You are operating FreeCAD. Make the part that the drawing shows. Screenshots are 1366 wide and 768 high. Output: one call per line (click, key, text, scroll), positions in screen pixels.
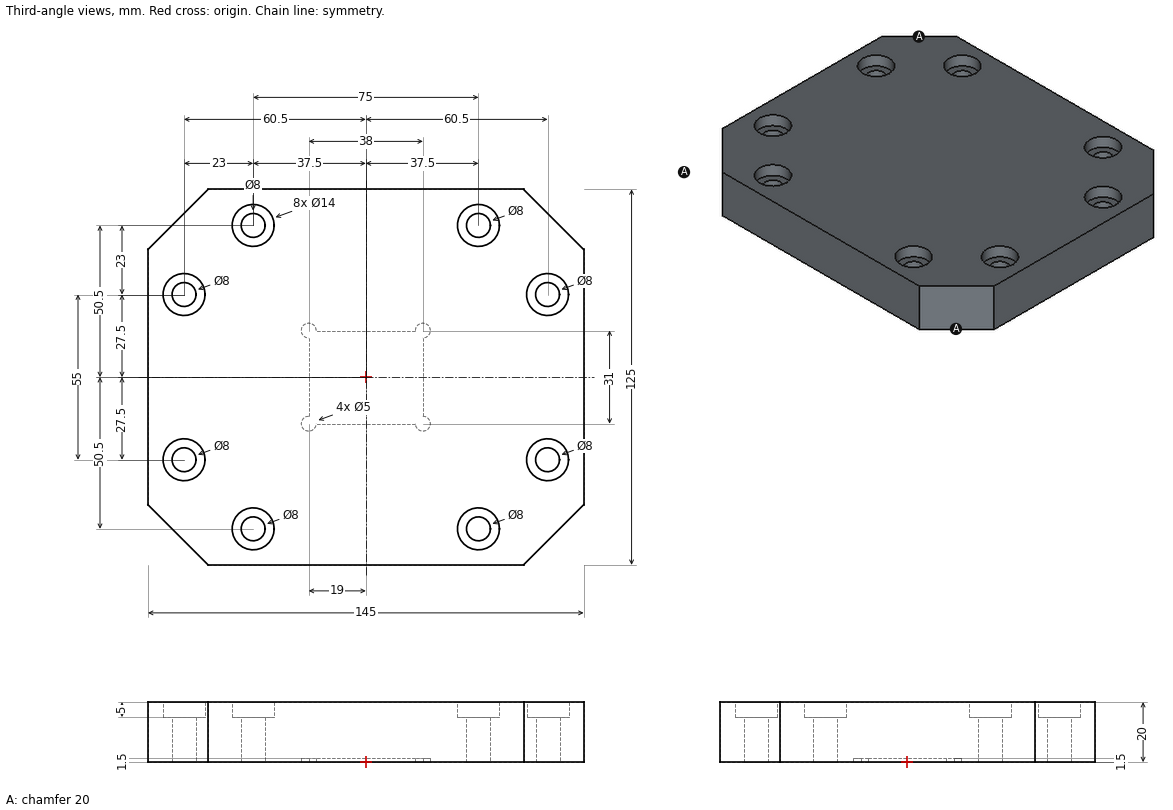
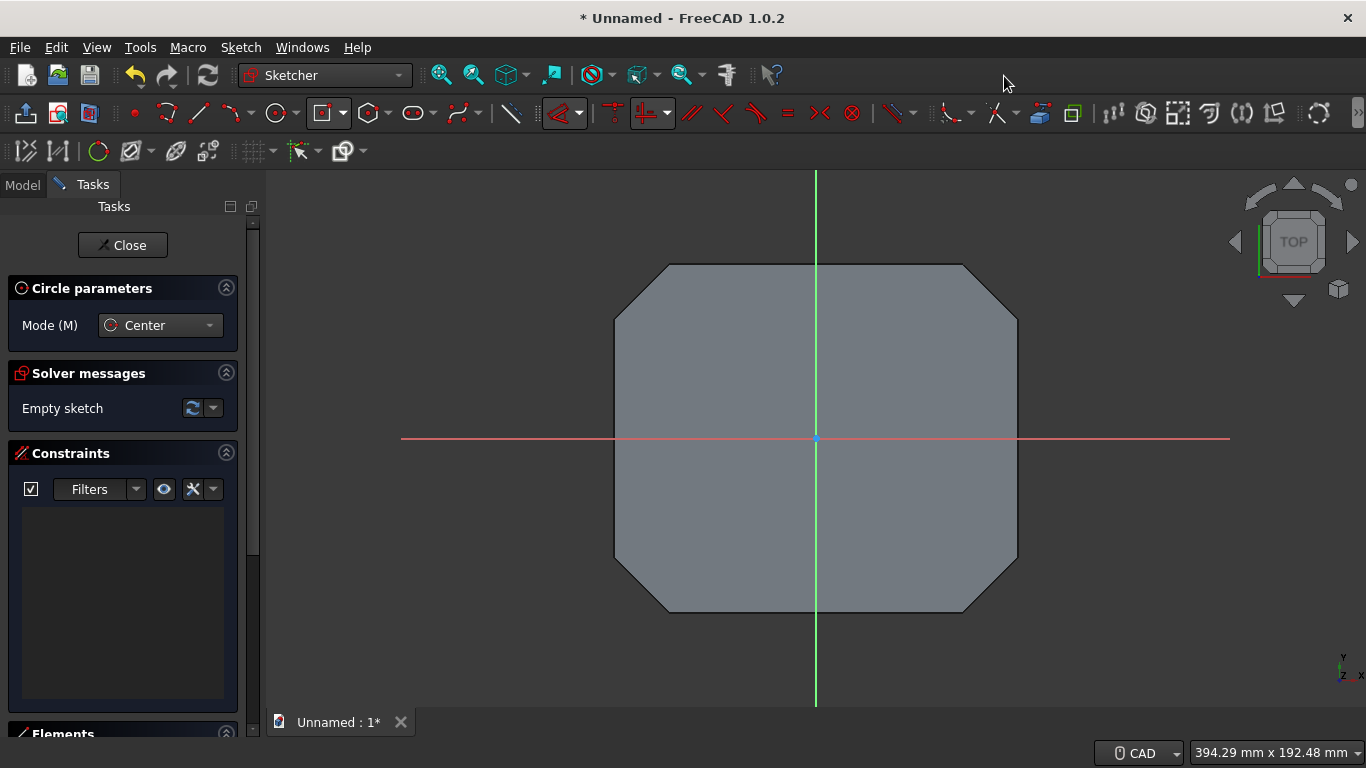
click(711, 298)
click(725, 284)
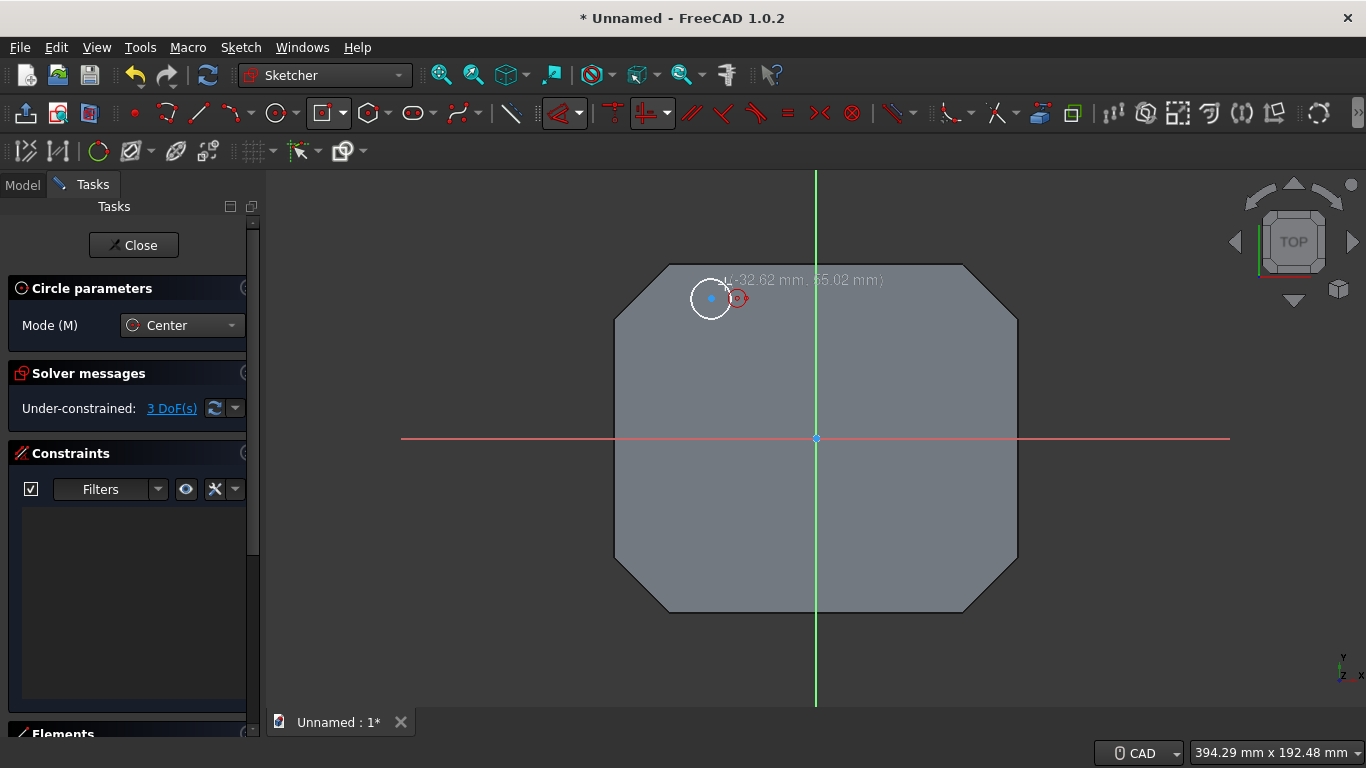
click(921, 298)
click(934, 284)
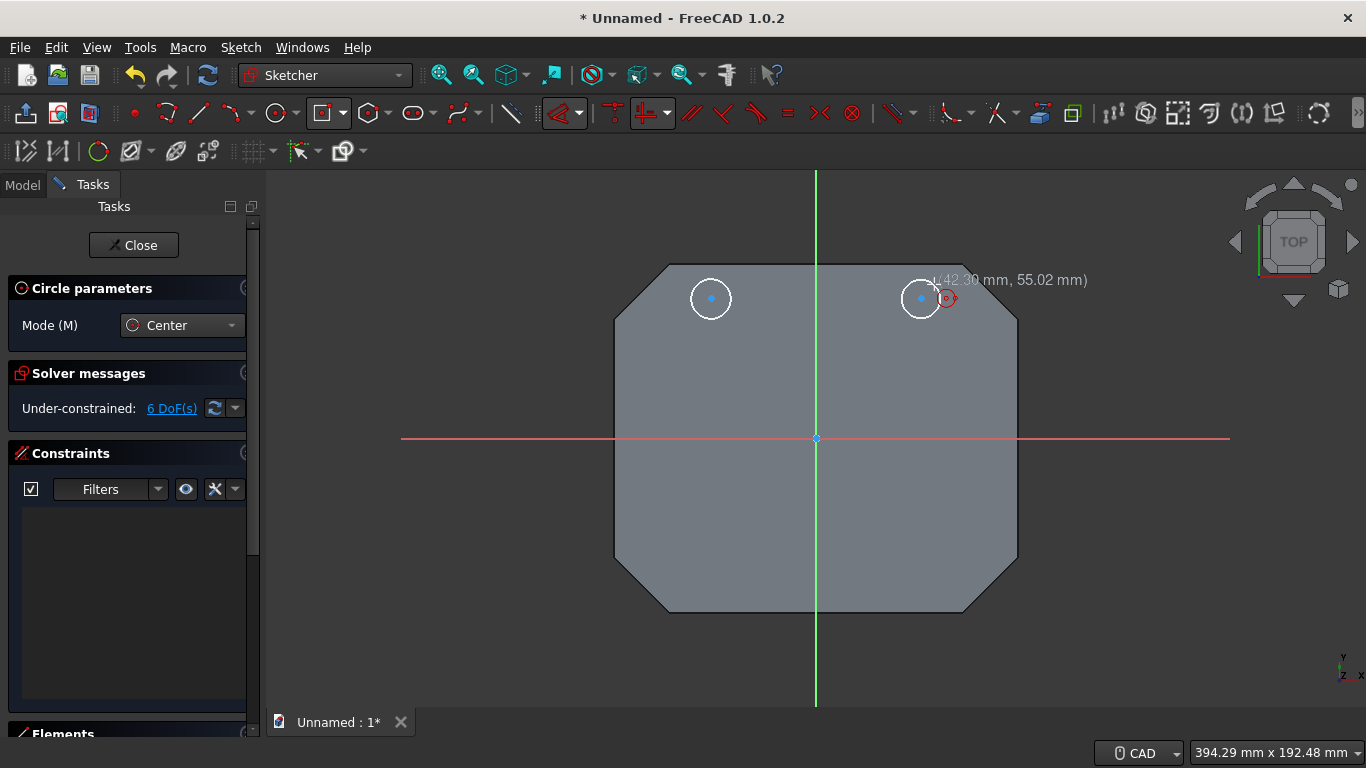
click(647, 362)
click(661, 348)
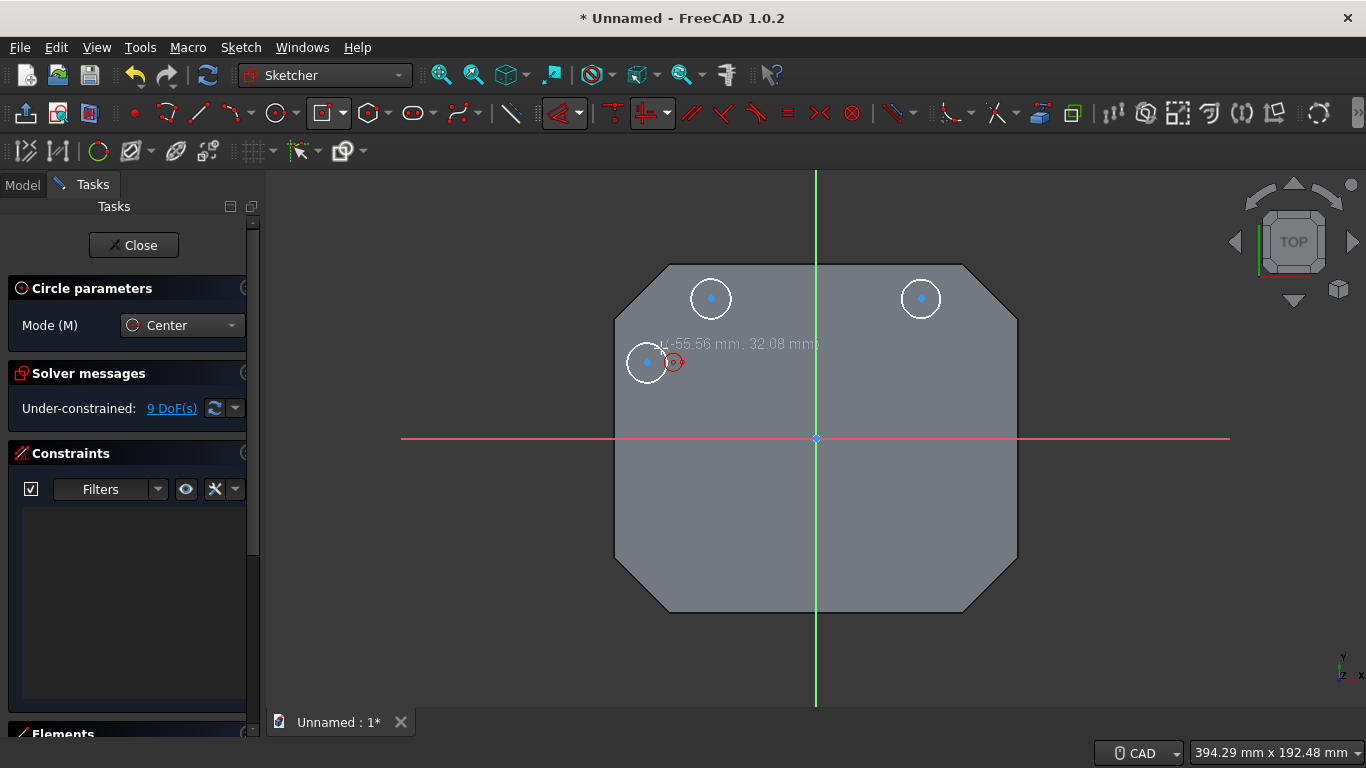
click(647, 515)
click(661, 501)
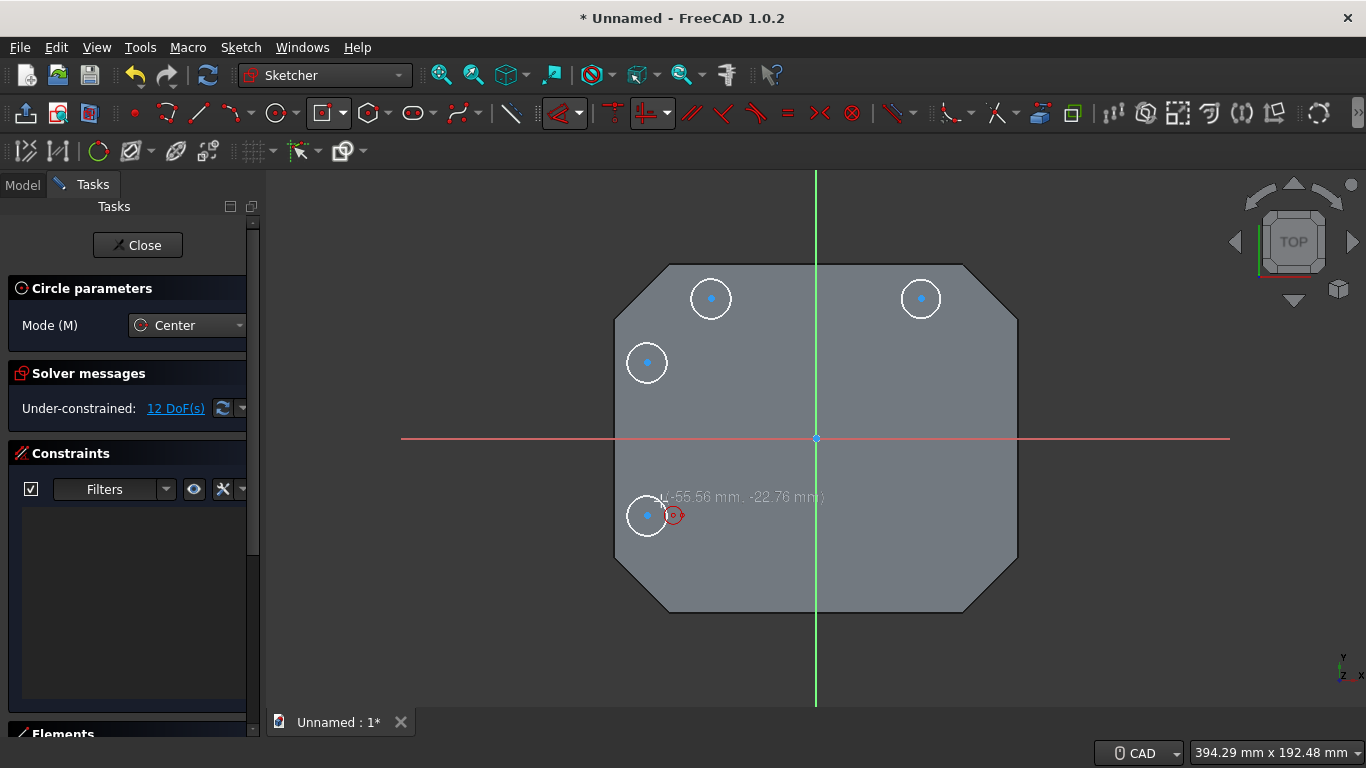
click(711, 579)
click(725, 566)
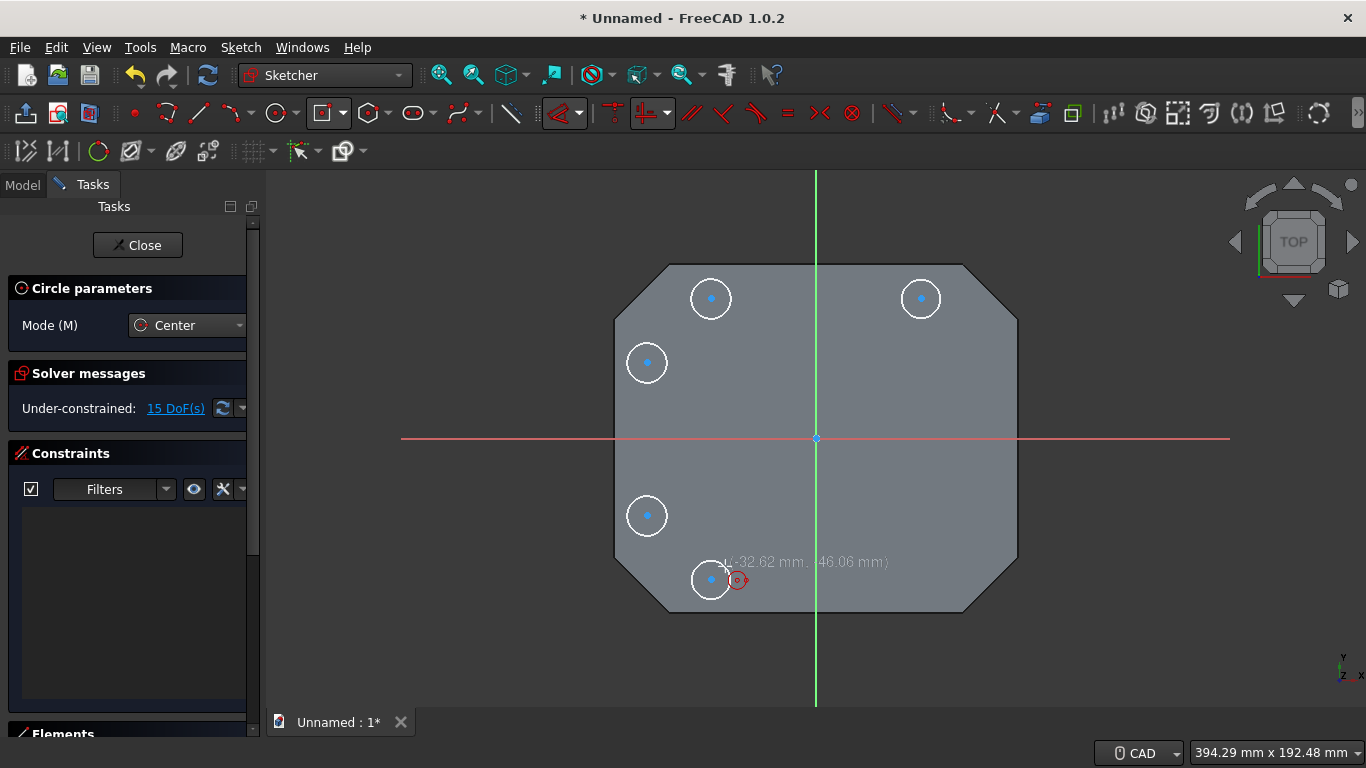
click(921, 579)
click(934, 566)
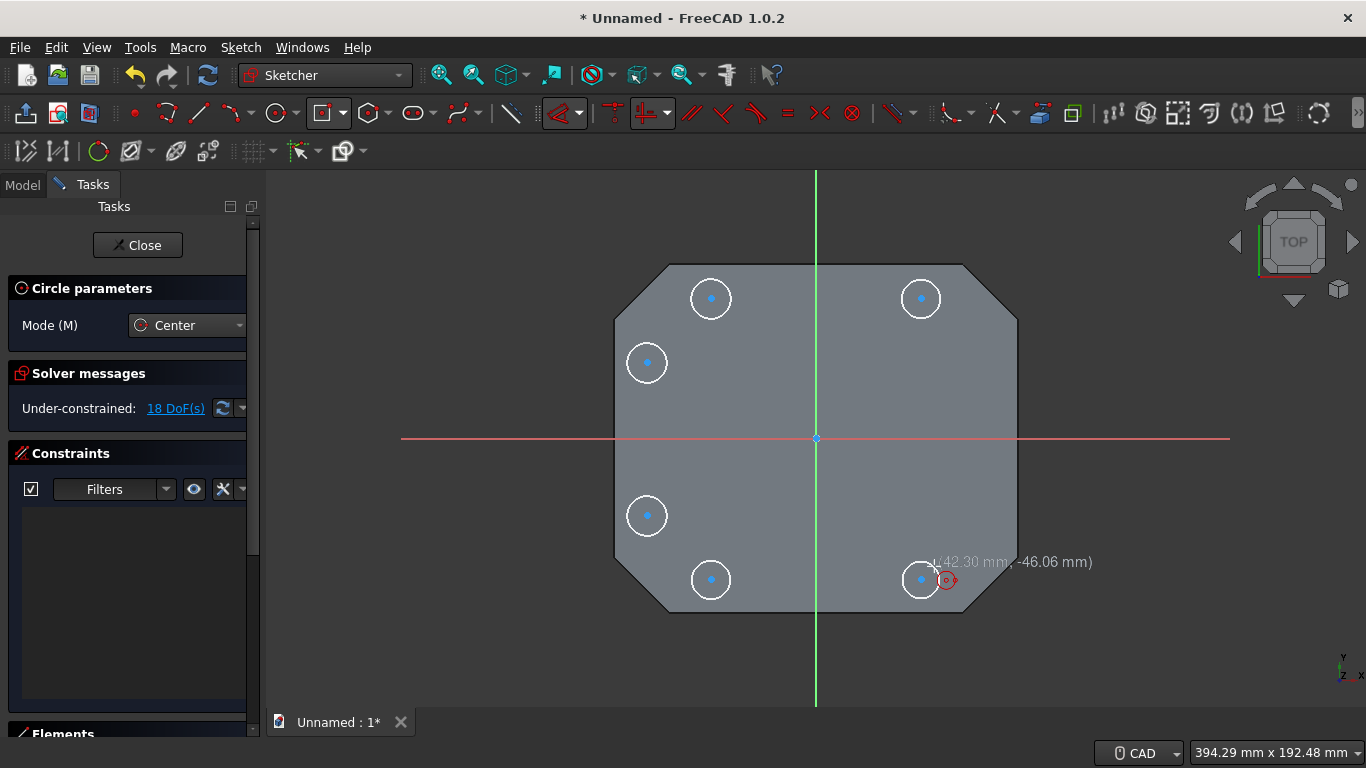
click(985, 362)
click(999, 348)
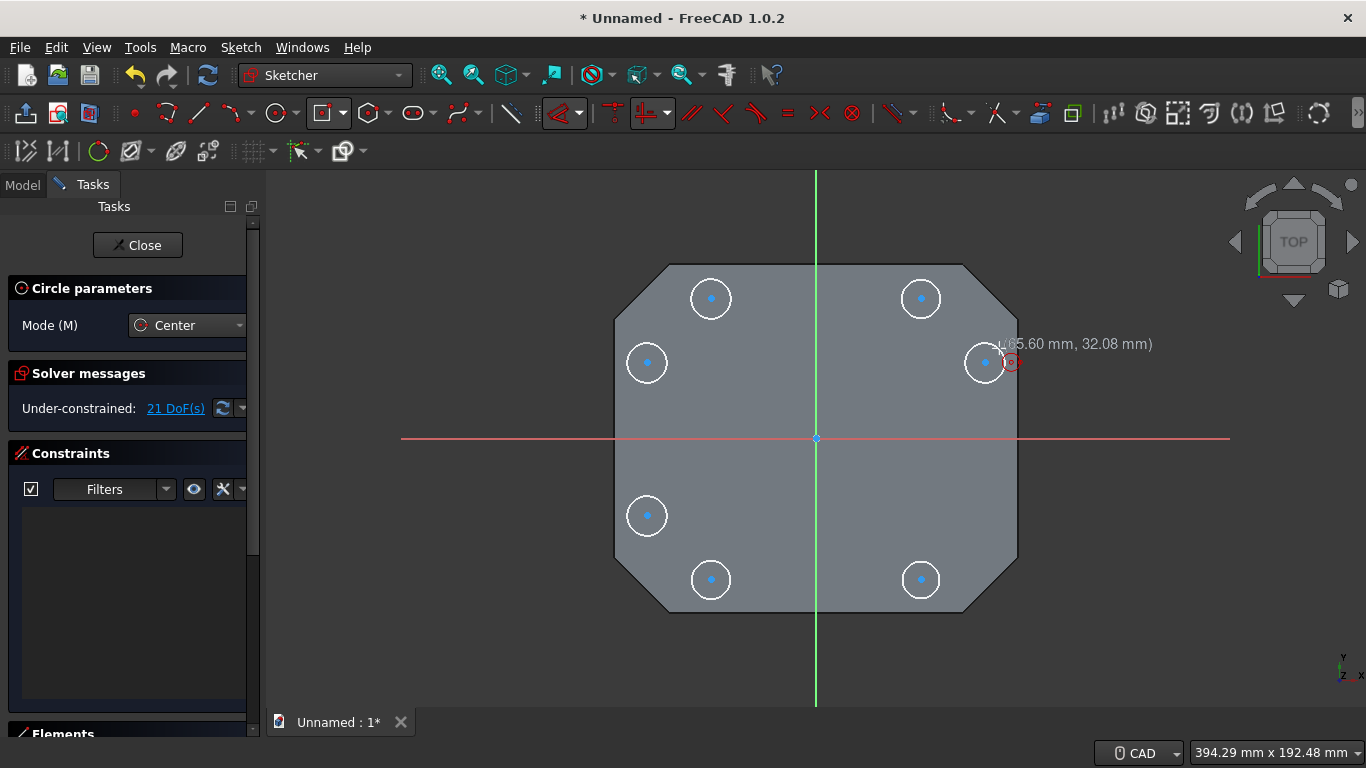
click(985, 515)
click(999, 501)
key(Escape)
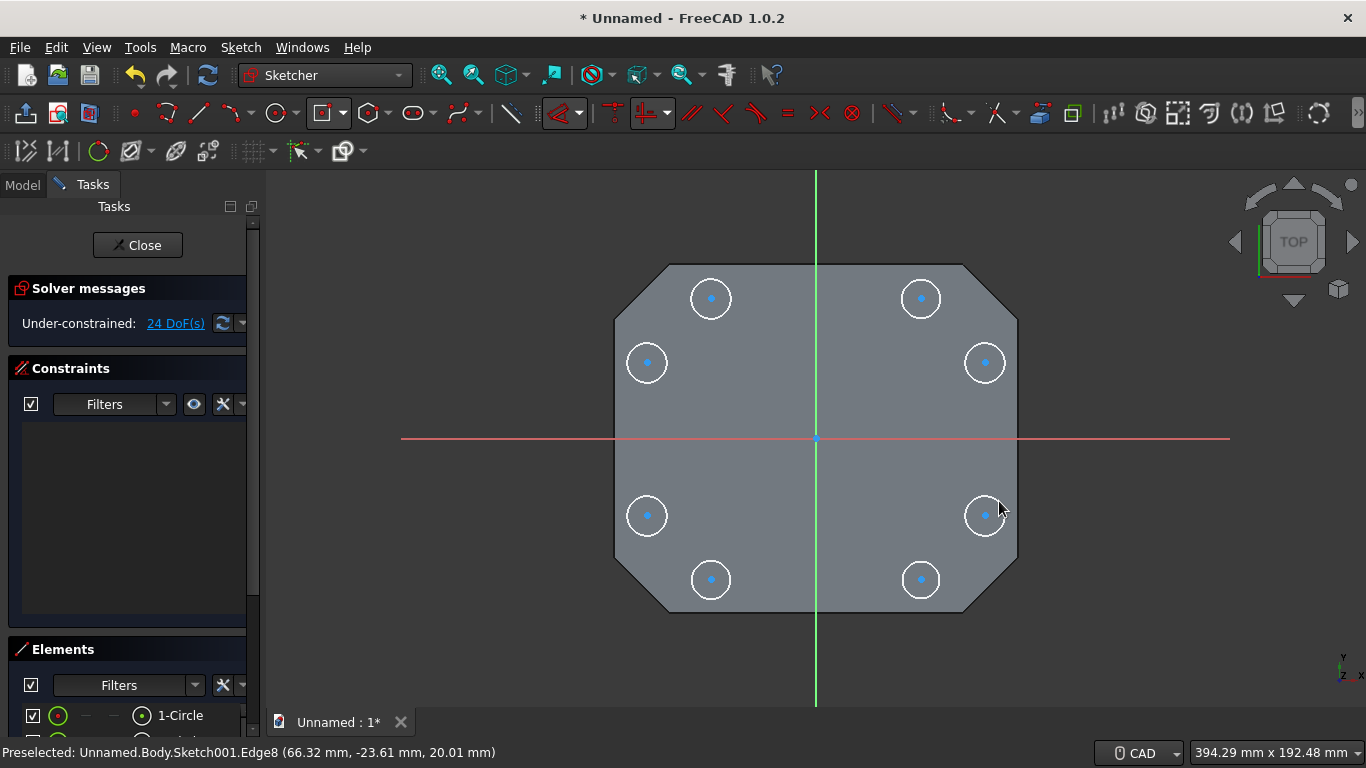
click(725, 285)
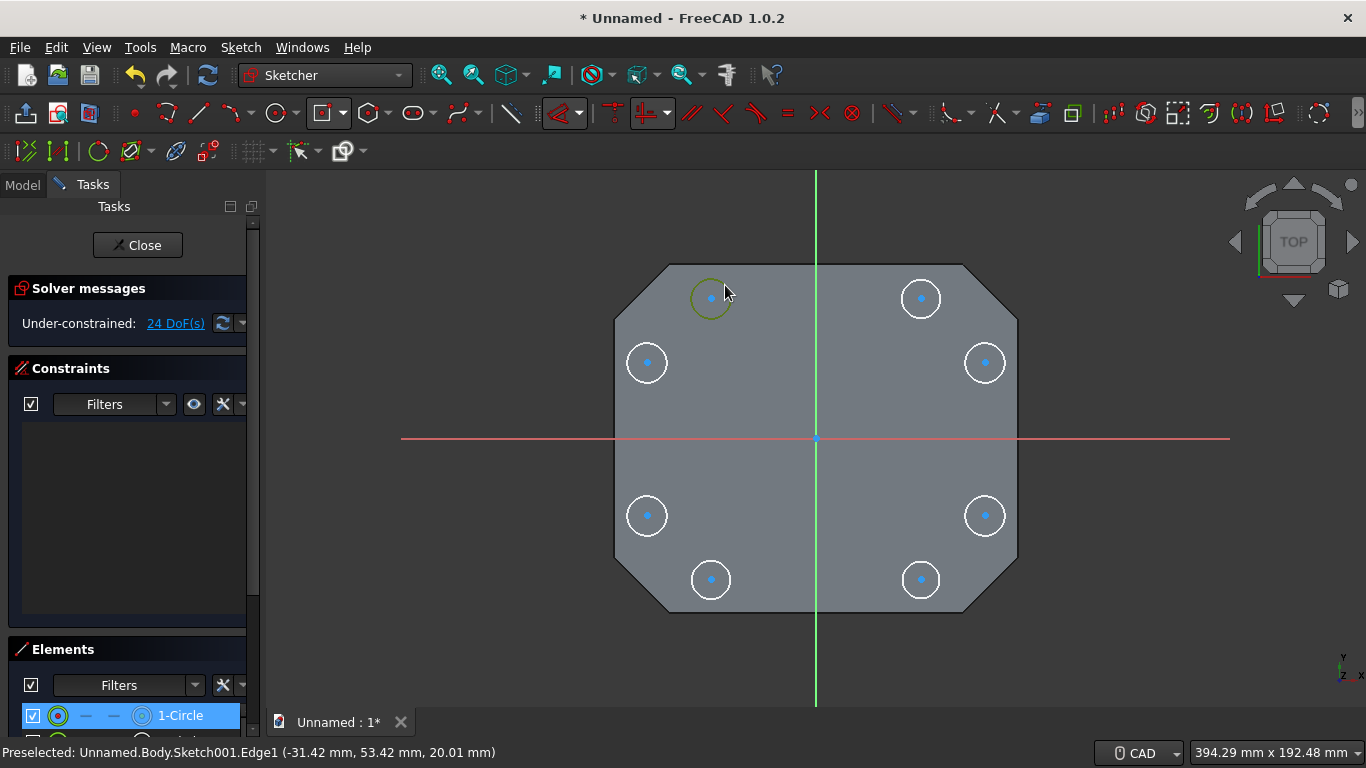
click(934, 285)